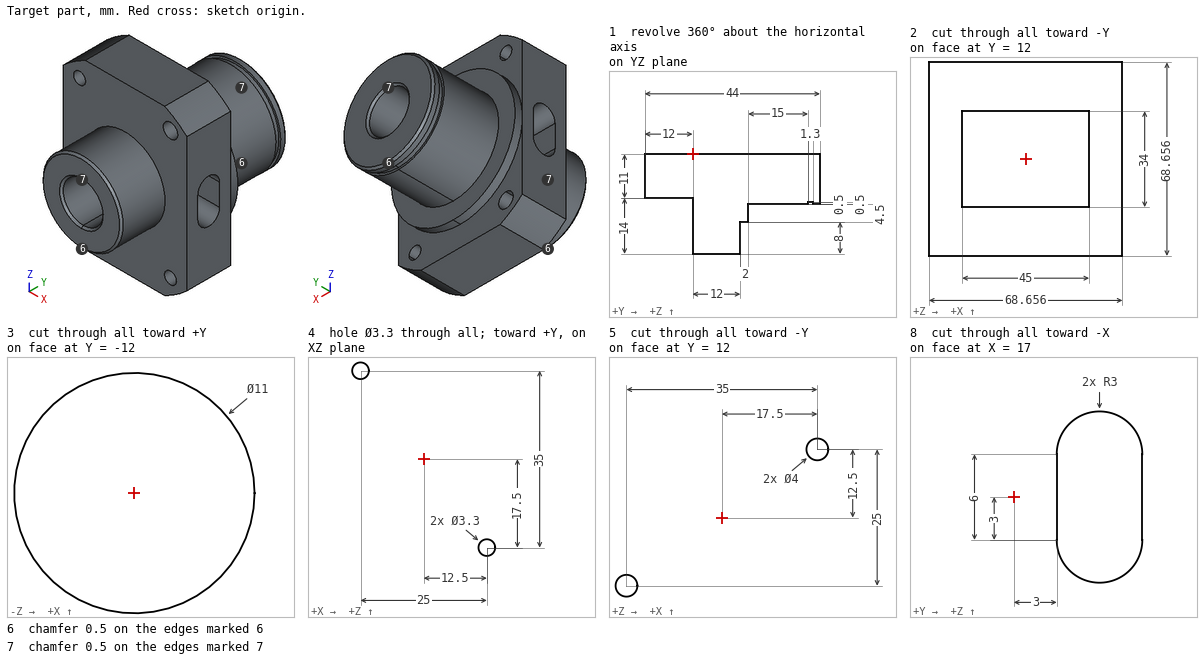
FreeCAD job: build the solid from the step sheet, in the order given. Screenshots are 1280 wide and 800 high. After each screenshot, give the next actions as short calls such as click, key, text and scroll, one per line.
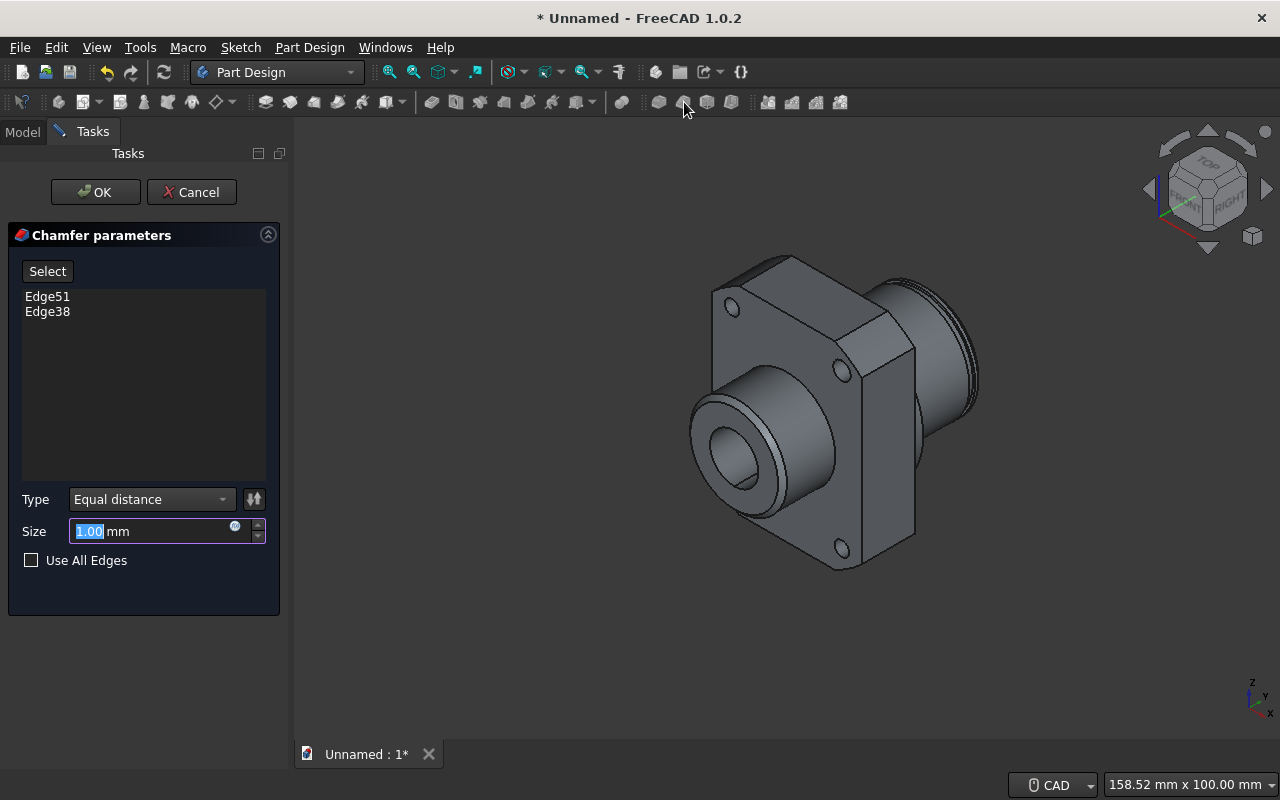
text(0.5)
key(Tab)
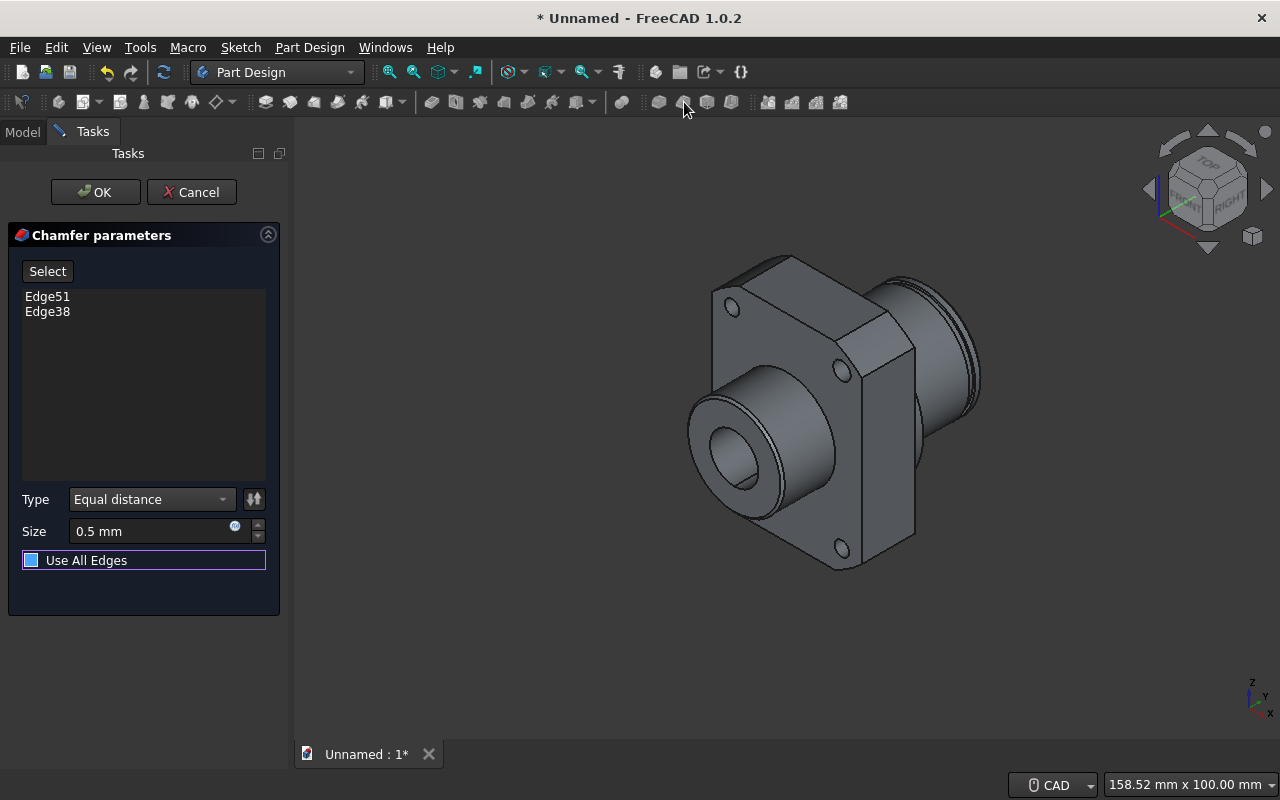
click(96, 192)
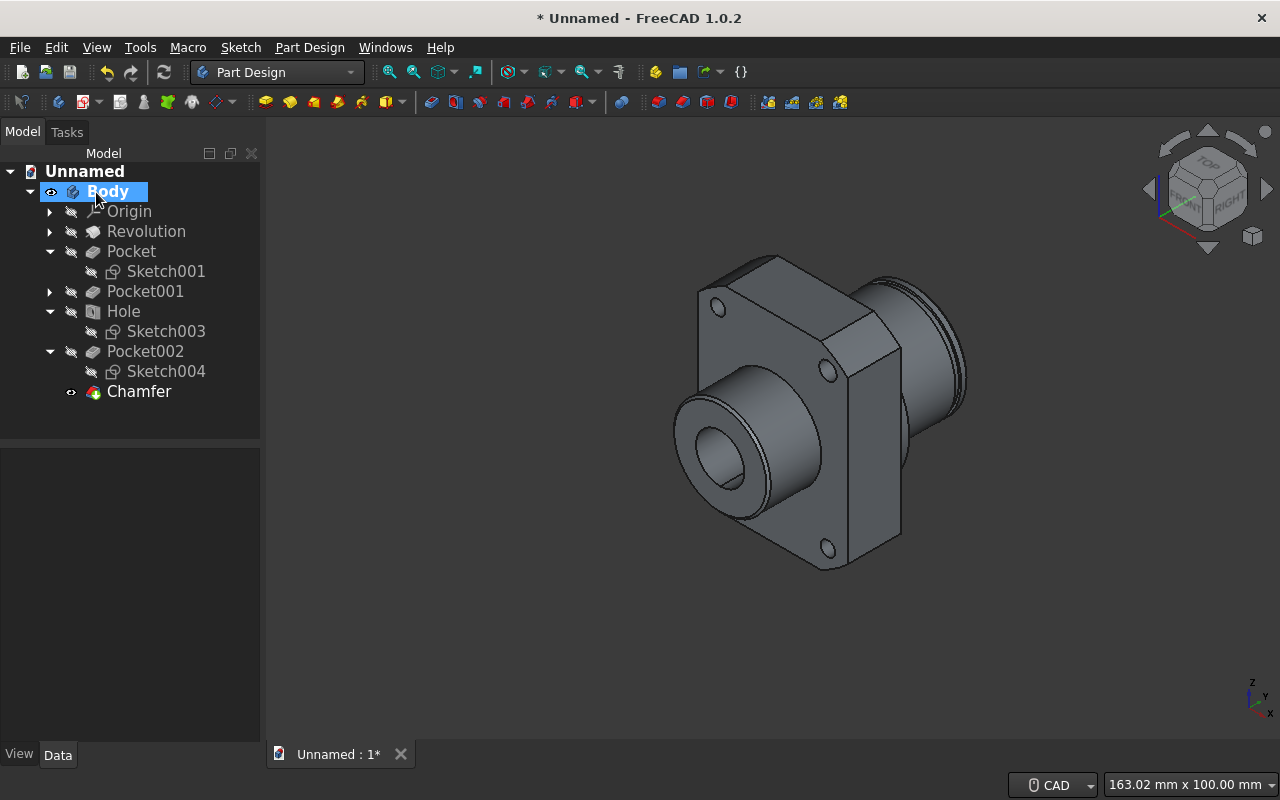
click(697, 436)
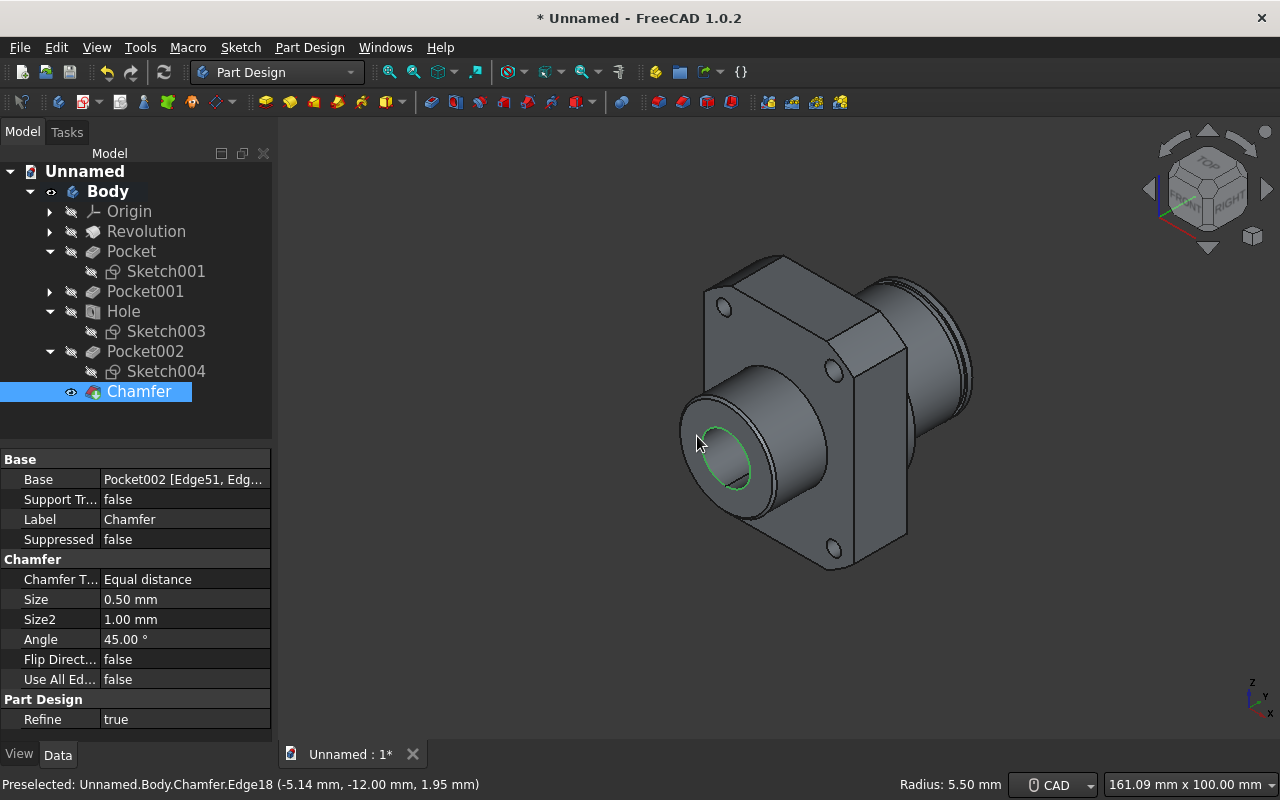
key(2)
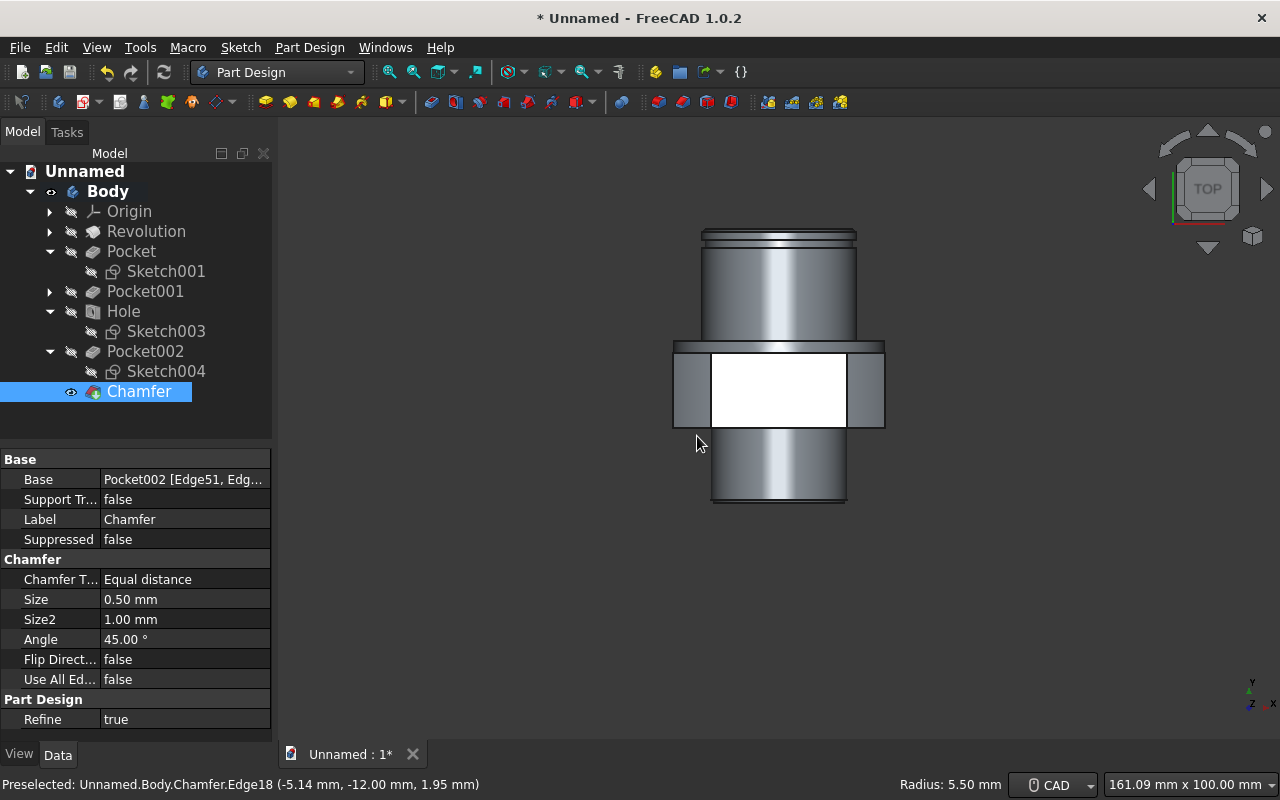
click(390, 72)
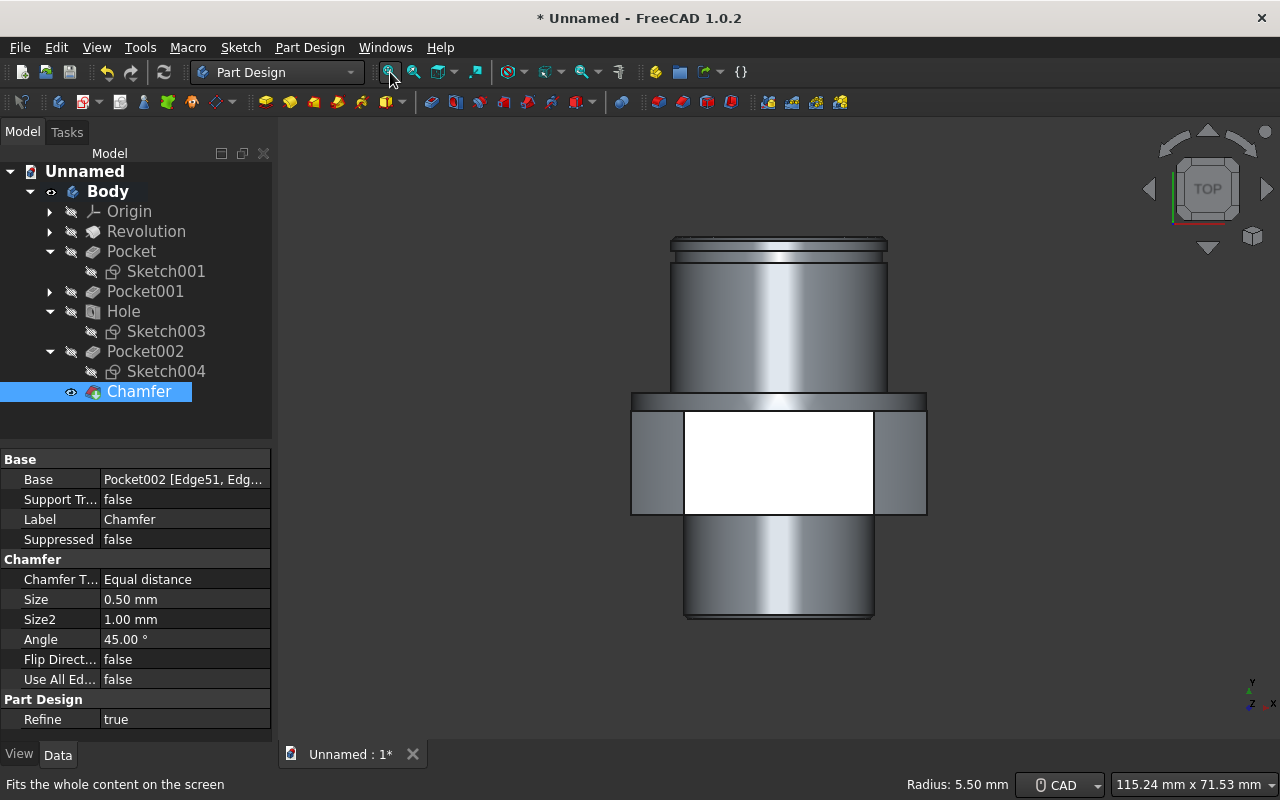
key(0)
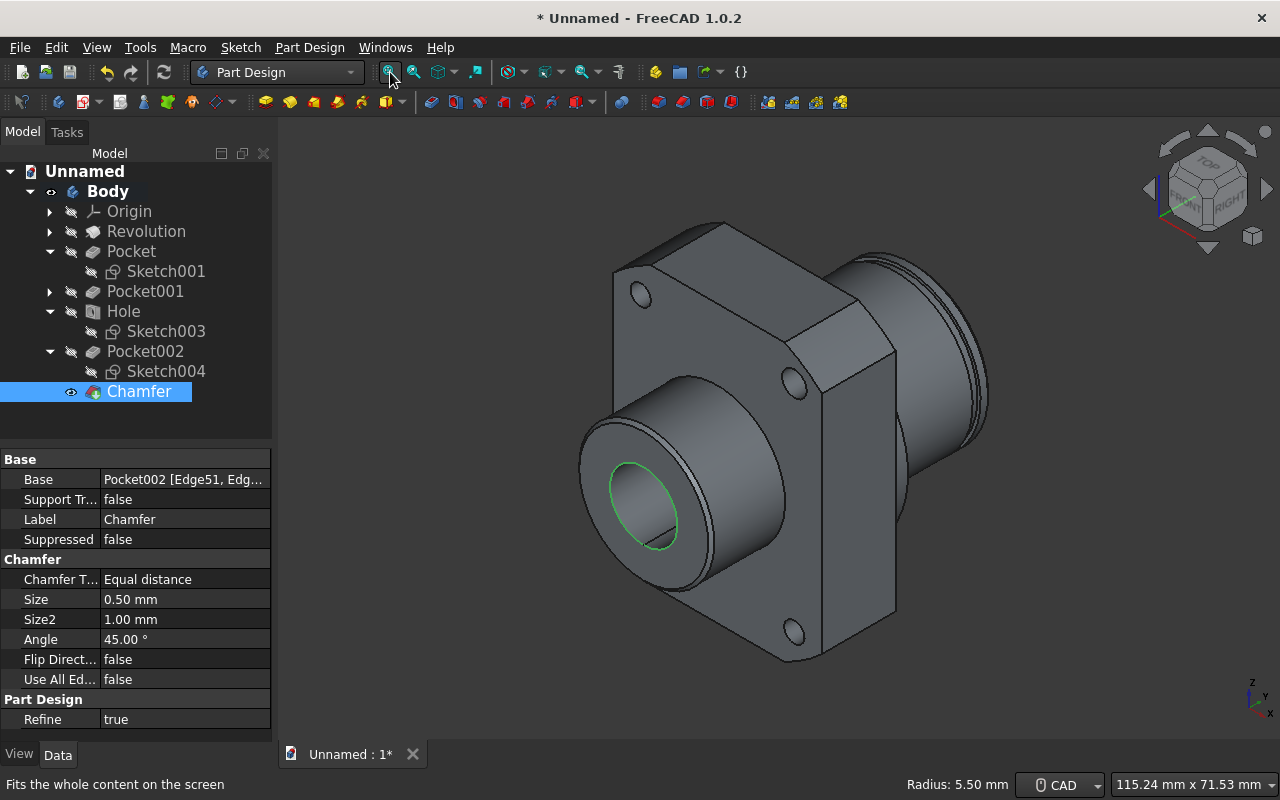
key(1)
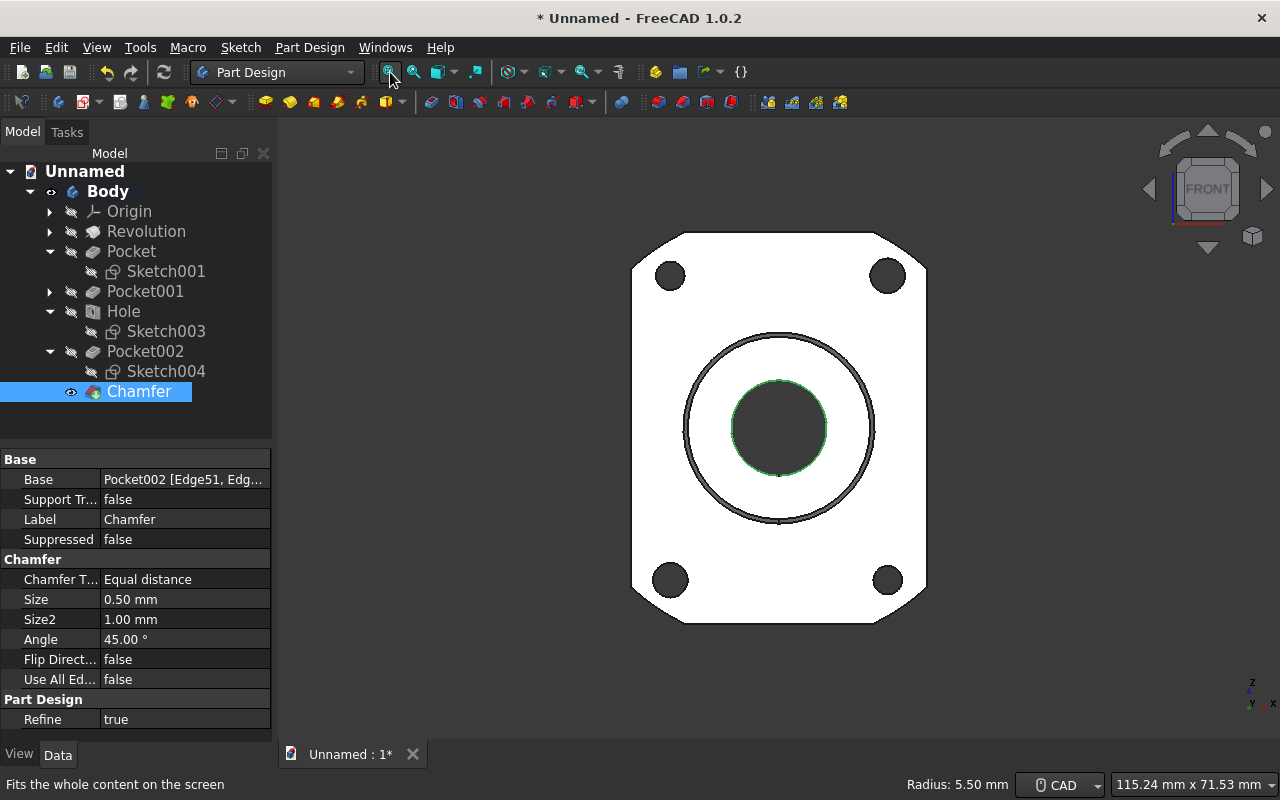
key(3)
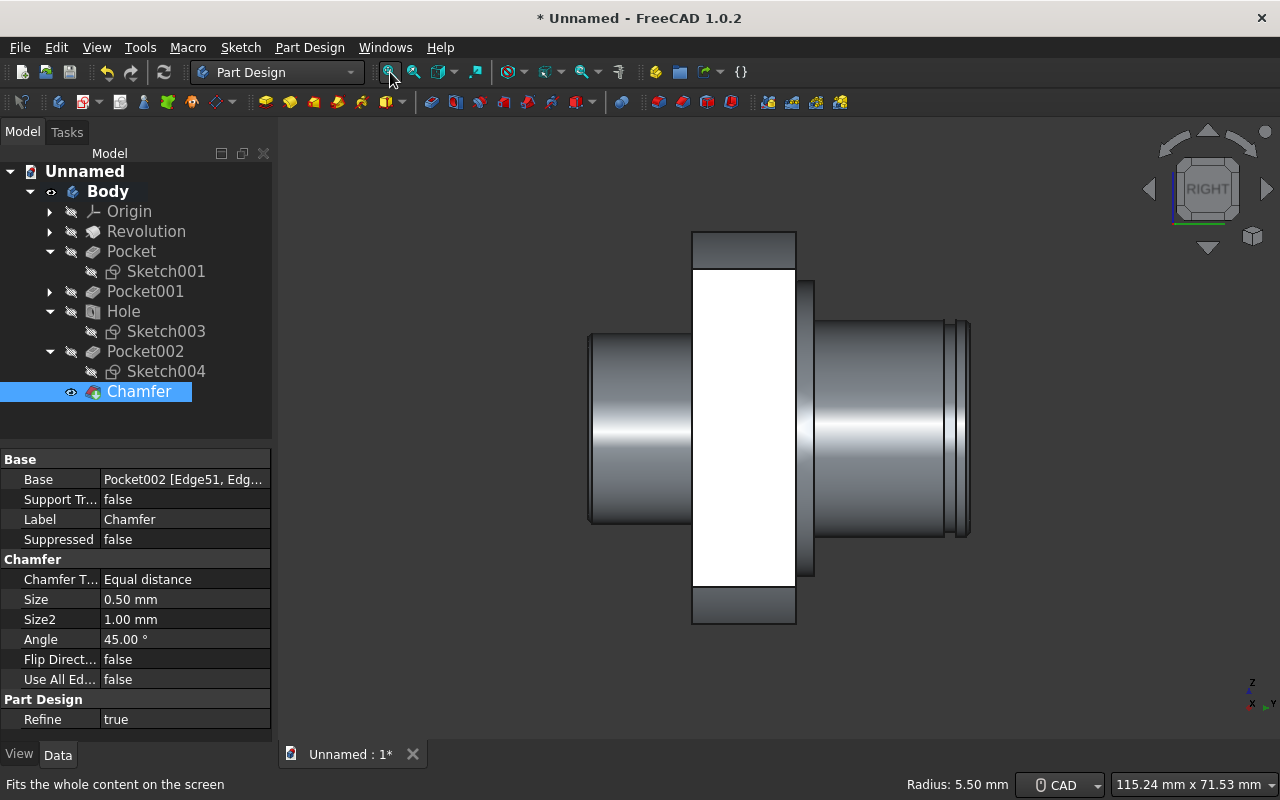
key(5)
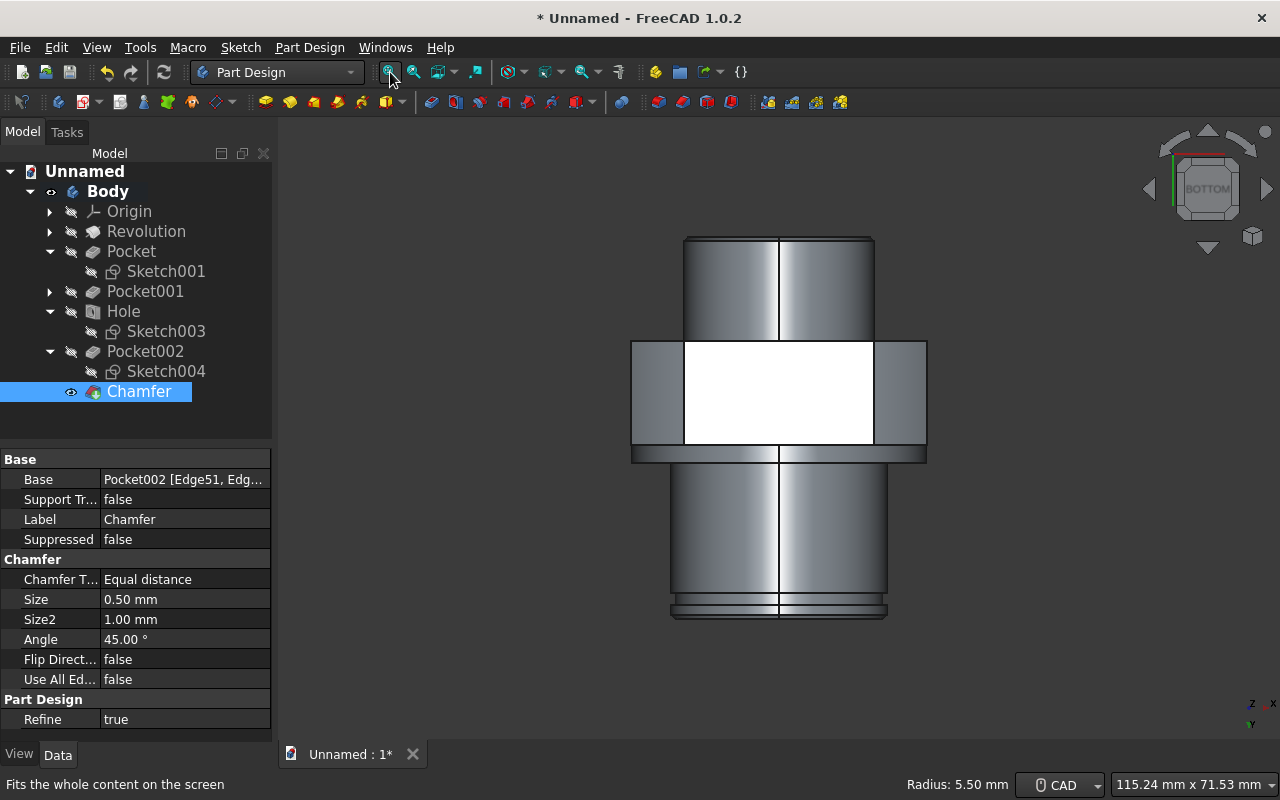
key(4)